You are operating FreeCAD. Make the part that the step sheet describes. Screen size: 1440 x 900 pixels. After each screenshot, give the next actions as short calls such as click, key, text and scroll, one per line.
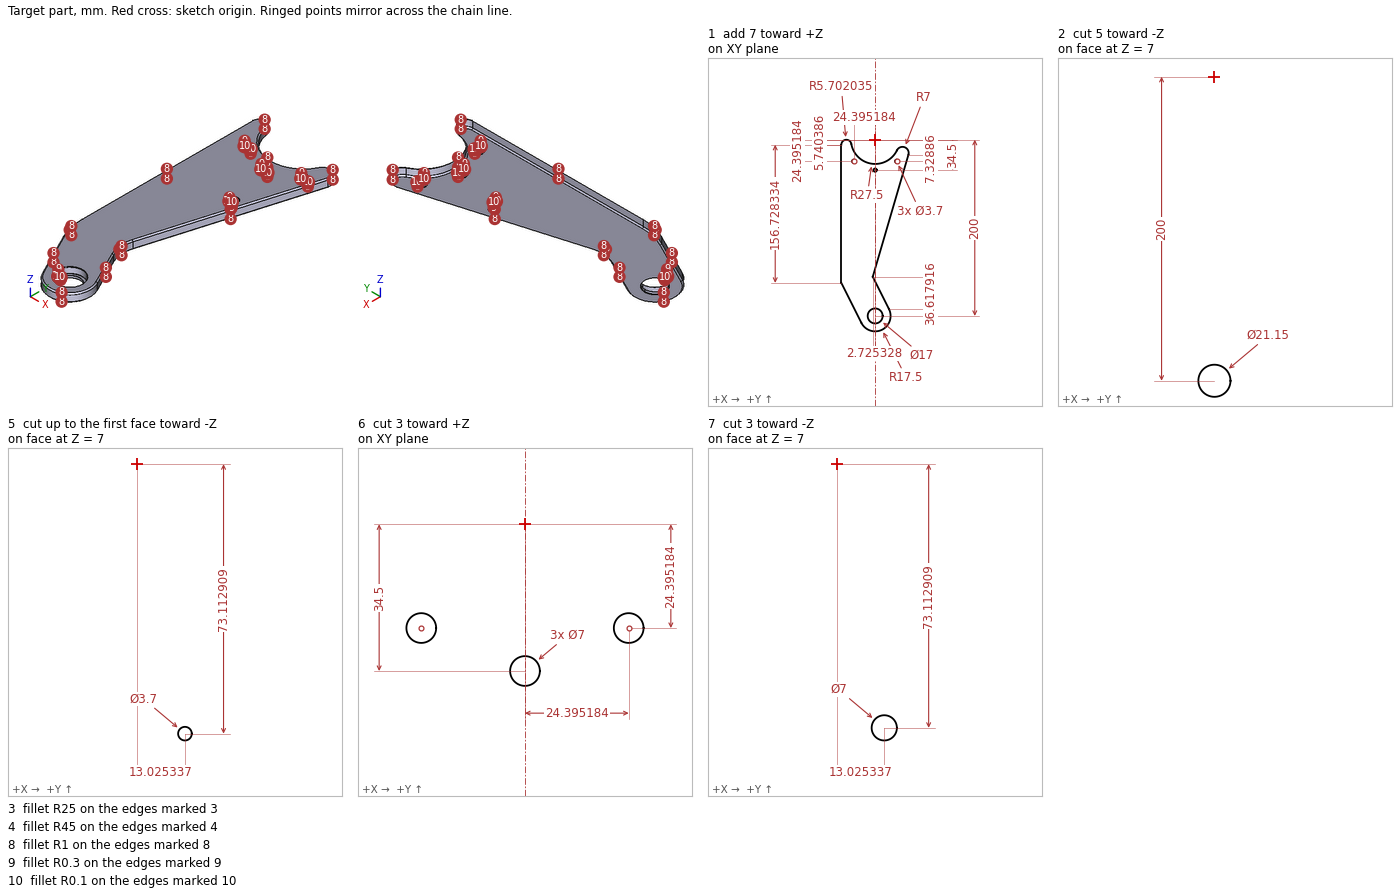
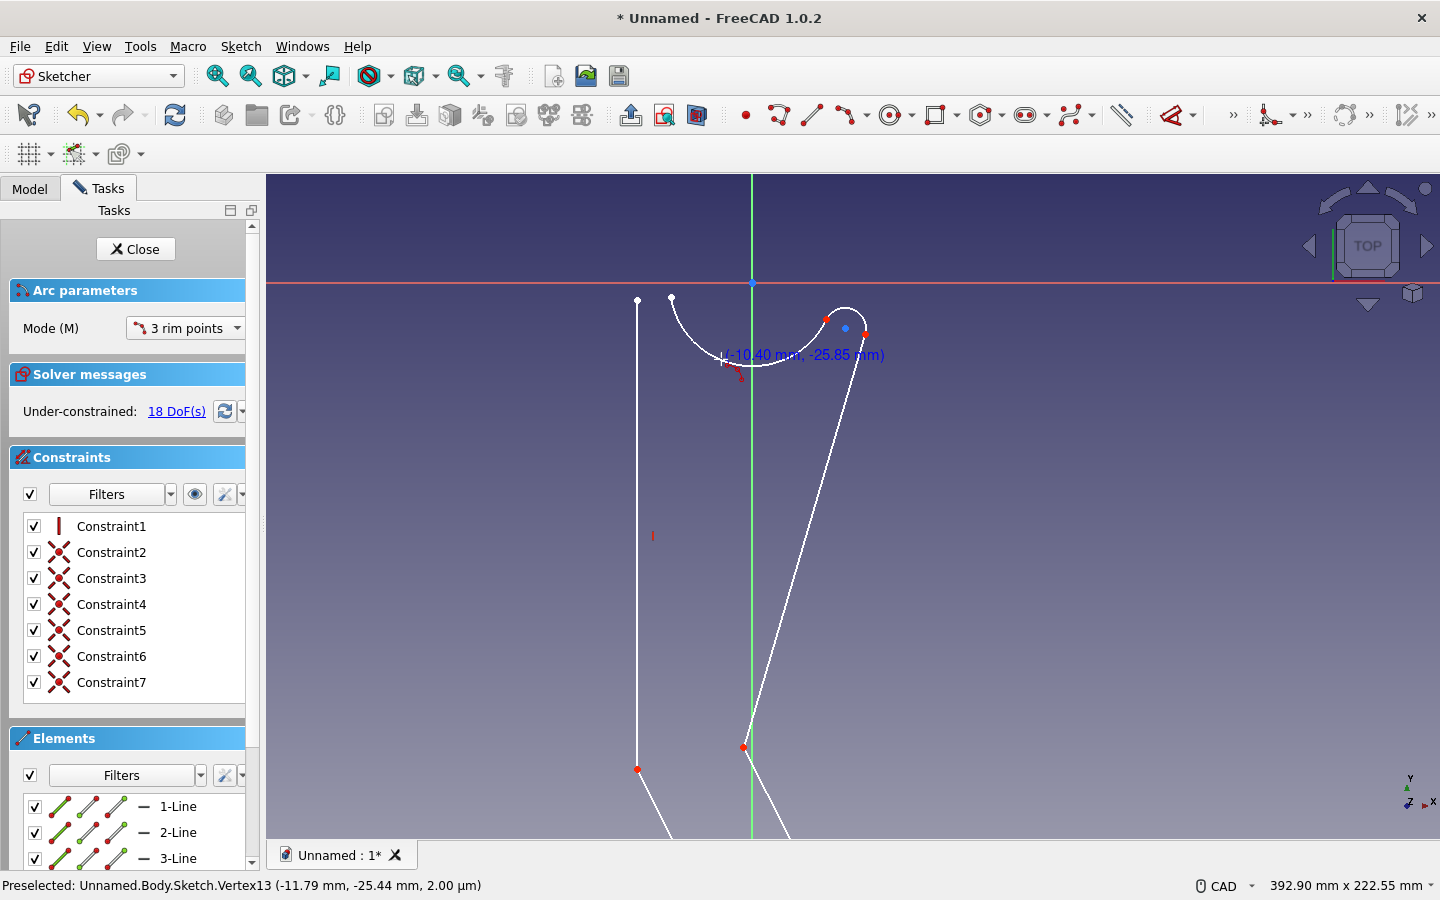
click(671, 298)
click(637, 301)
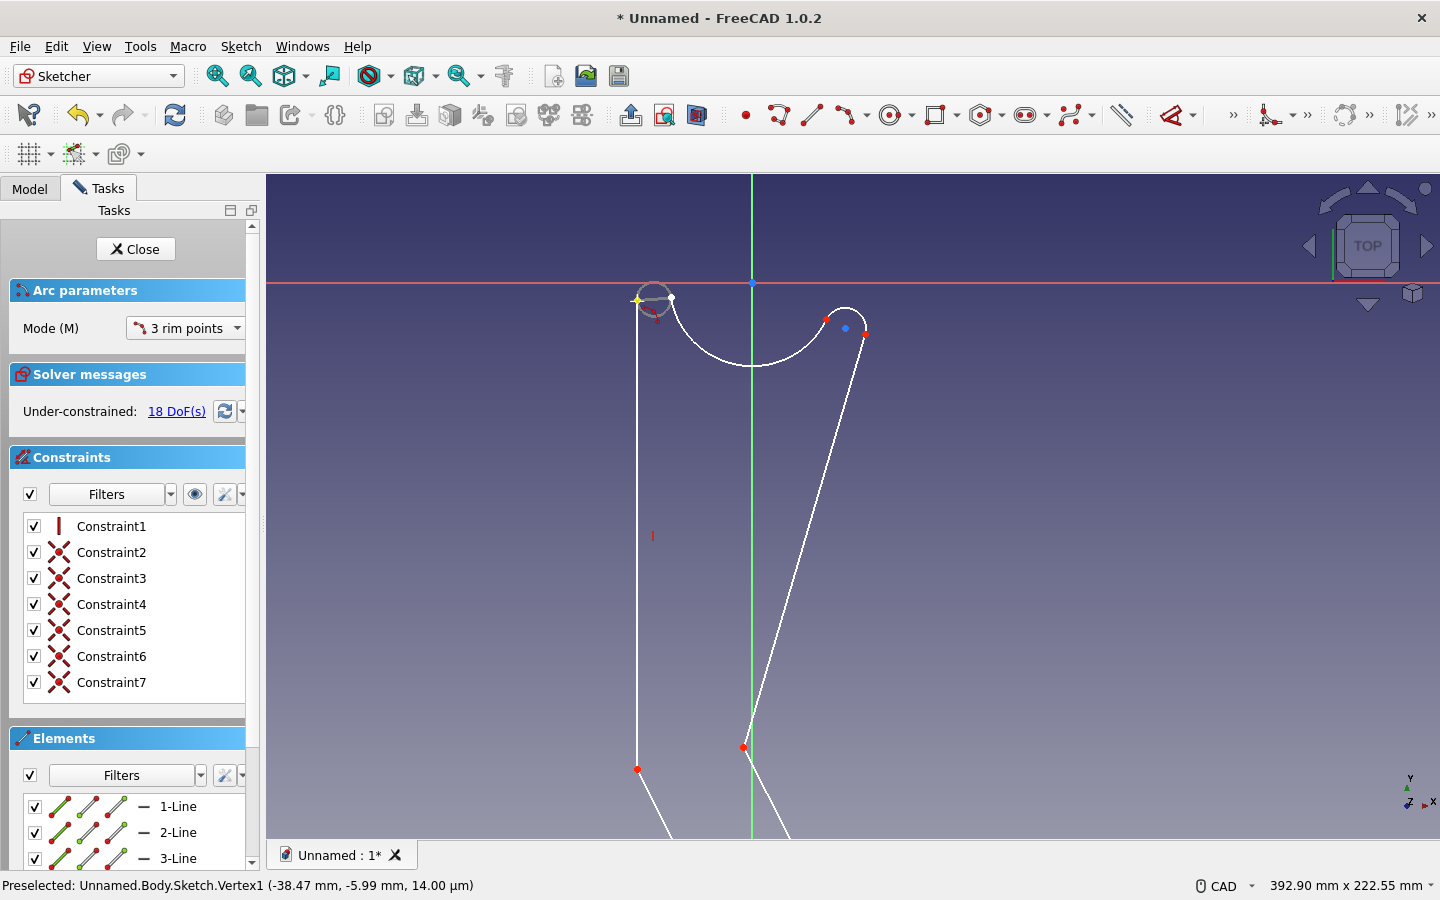
scroll(644, 287, up, 8)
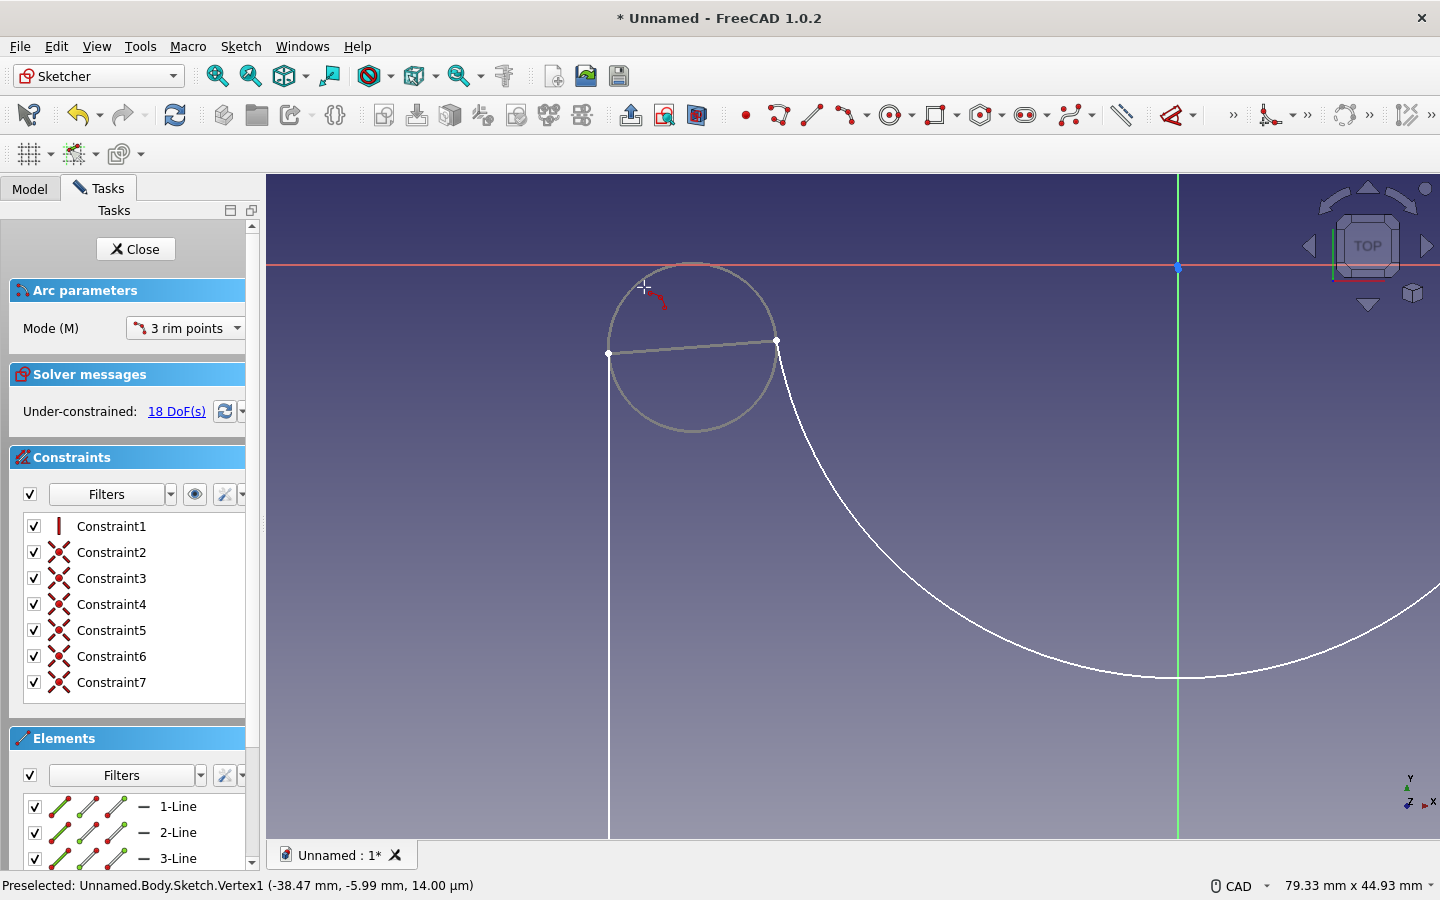
click(641, 285)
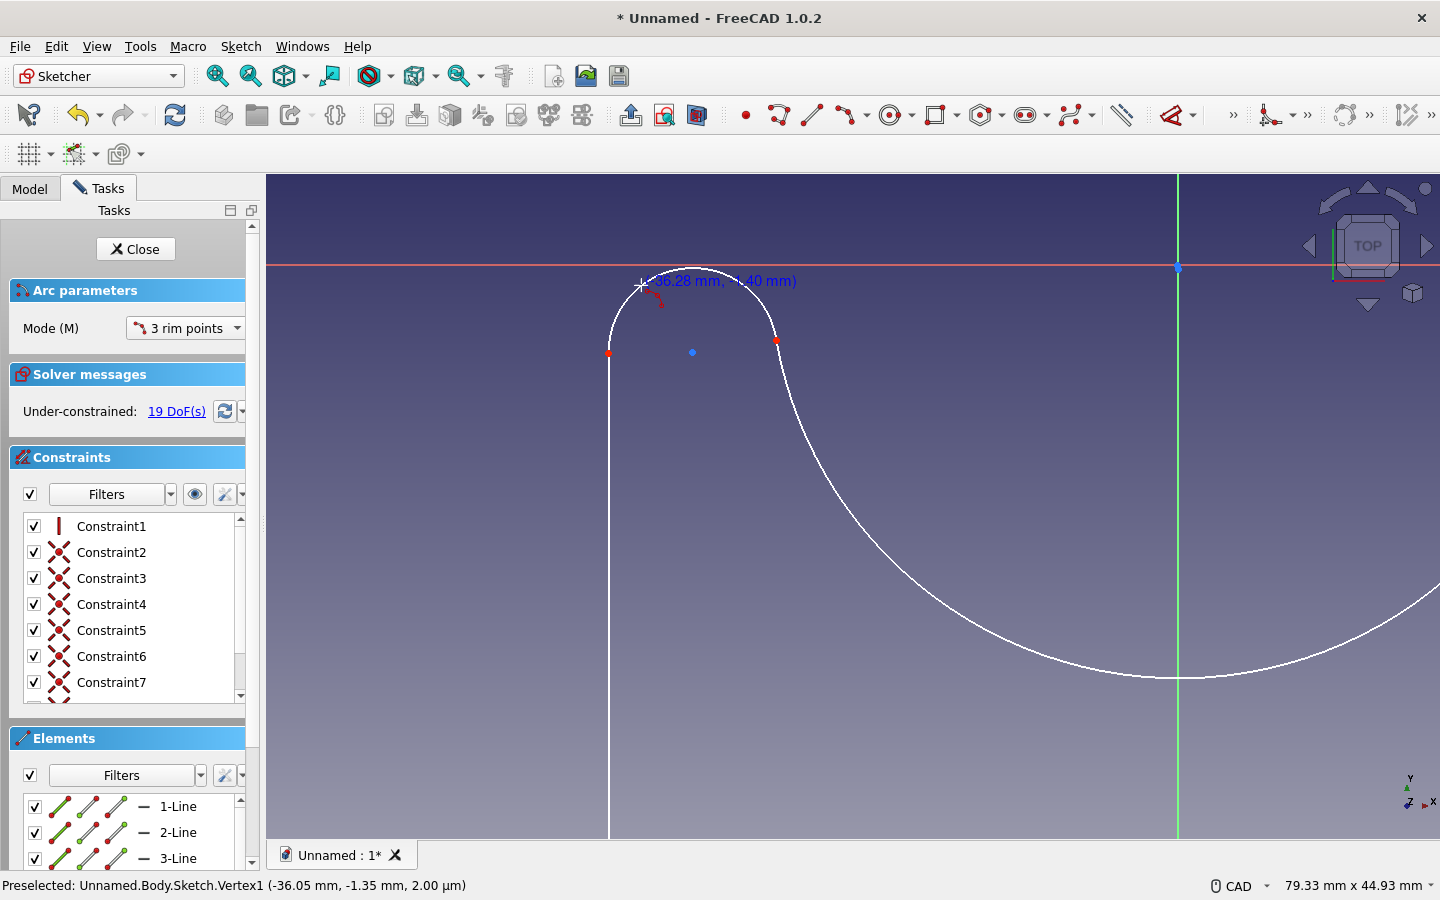
click(890, 116)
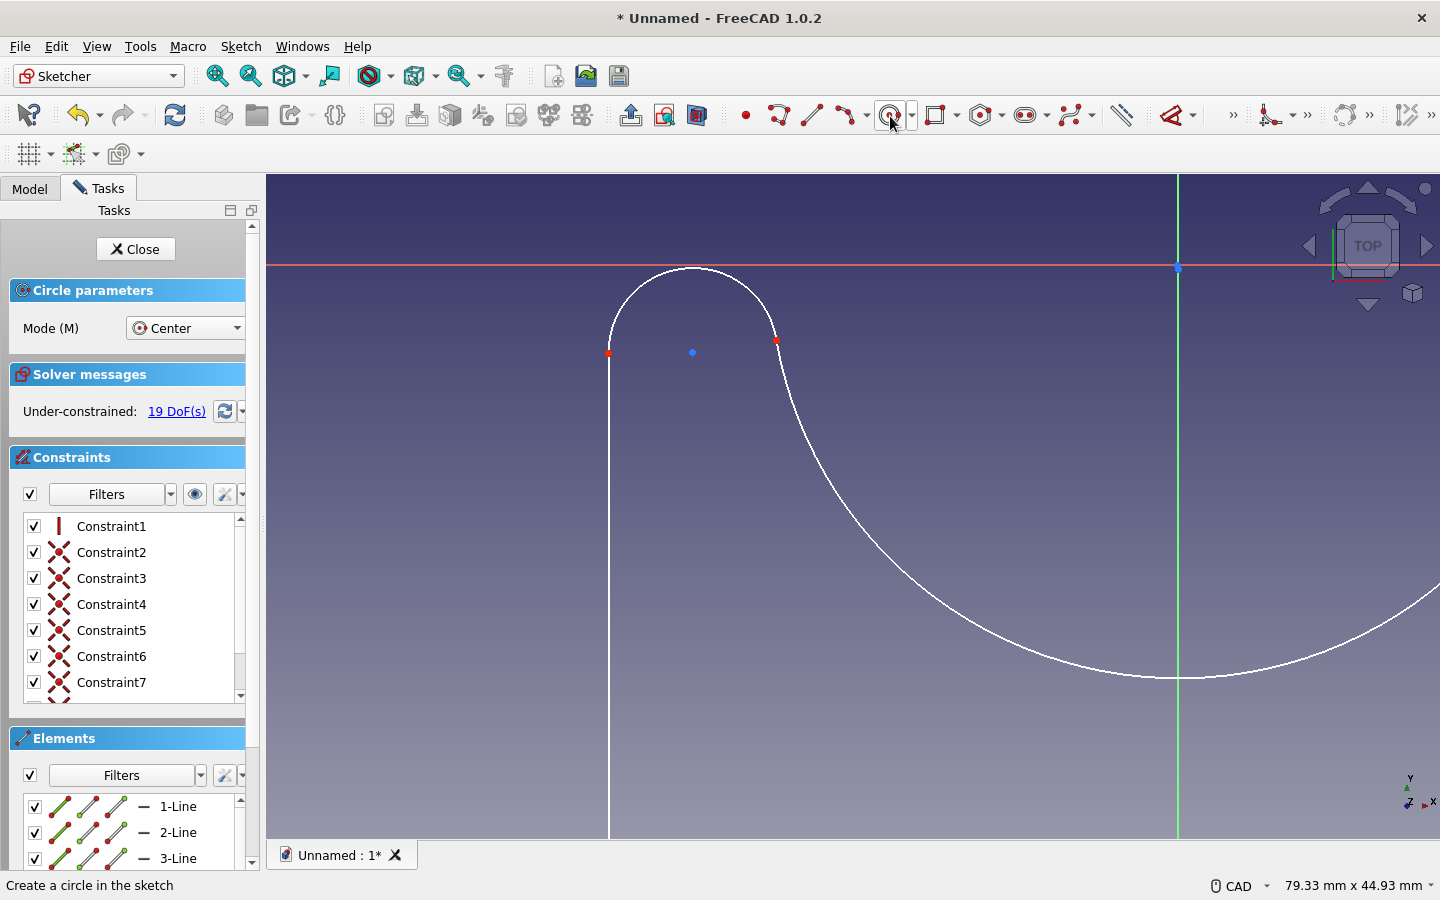
scroll(724, 294, down, 10)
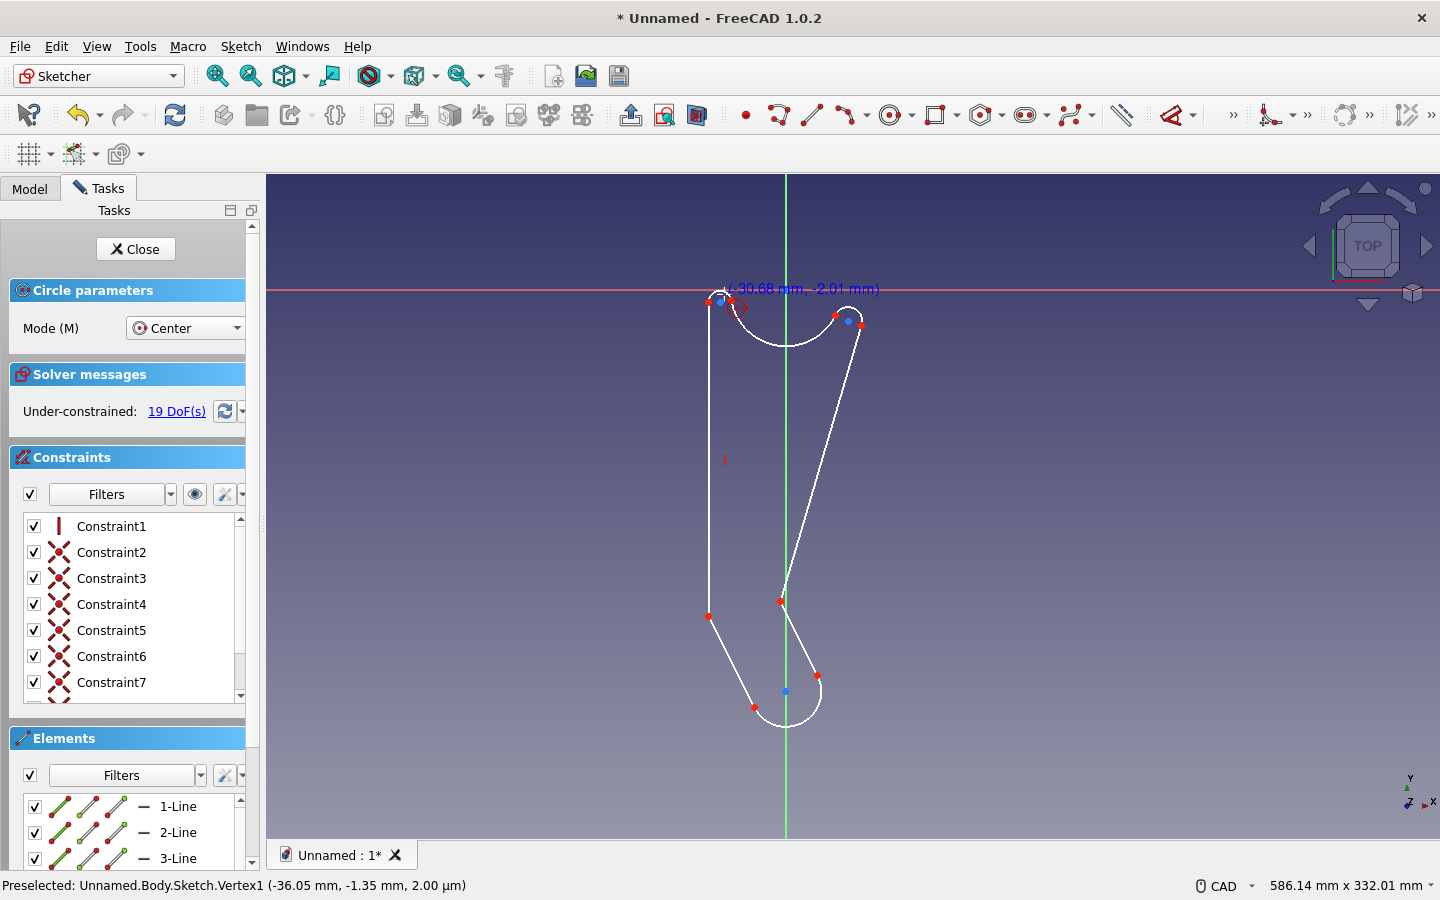
scroll(786, 691, up, 2)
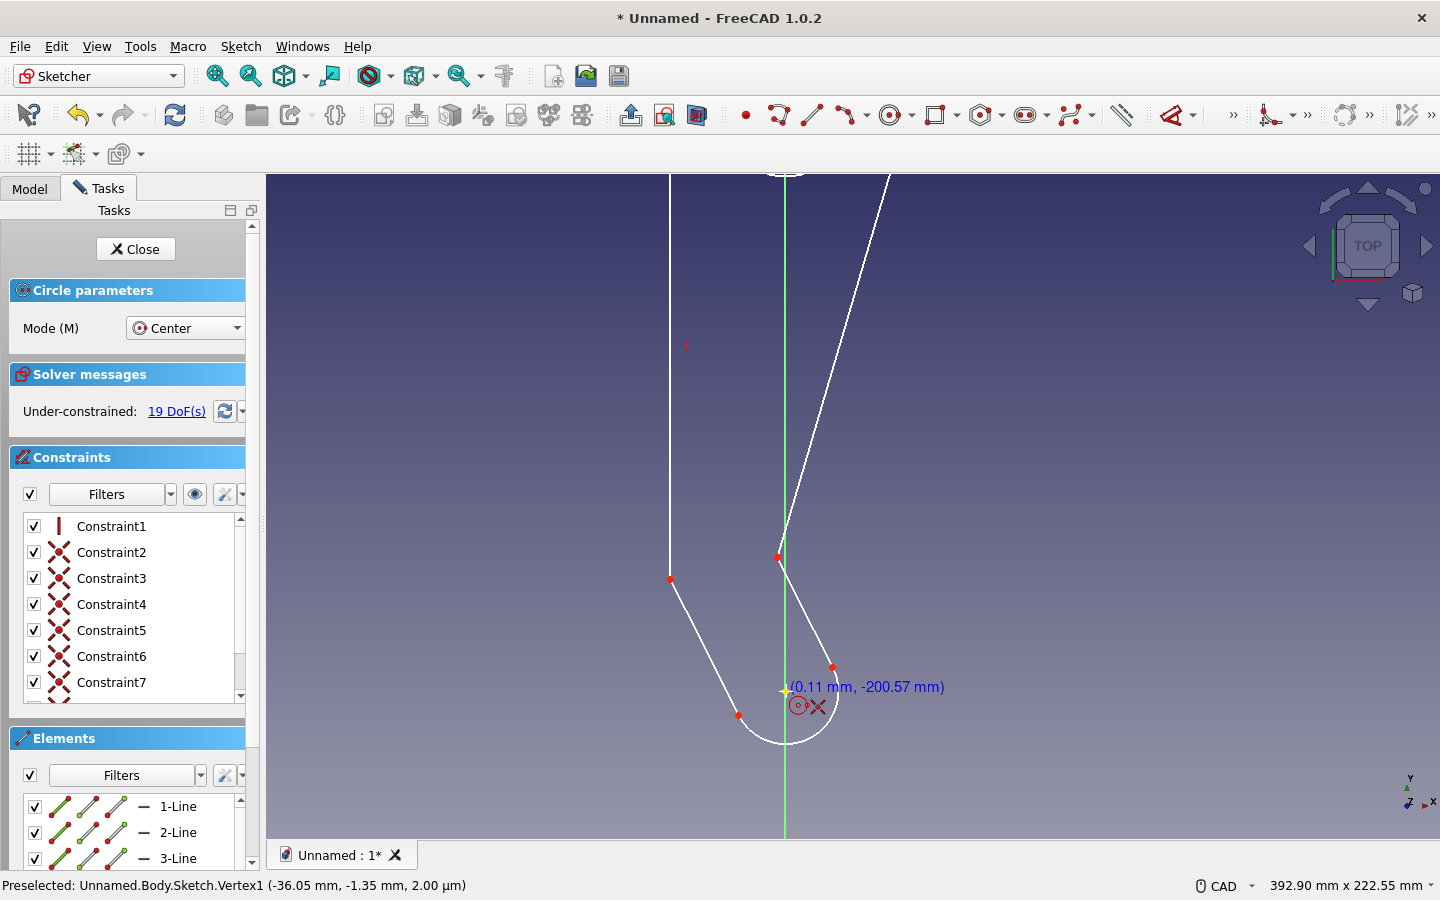
click(785, 690)
click(803, 672)